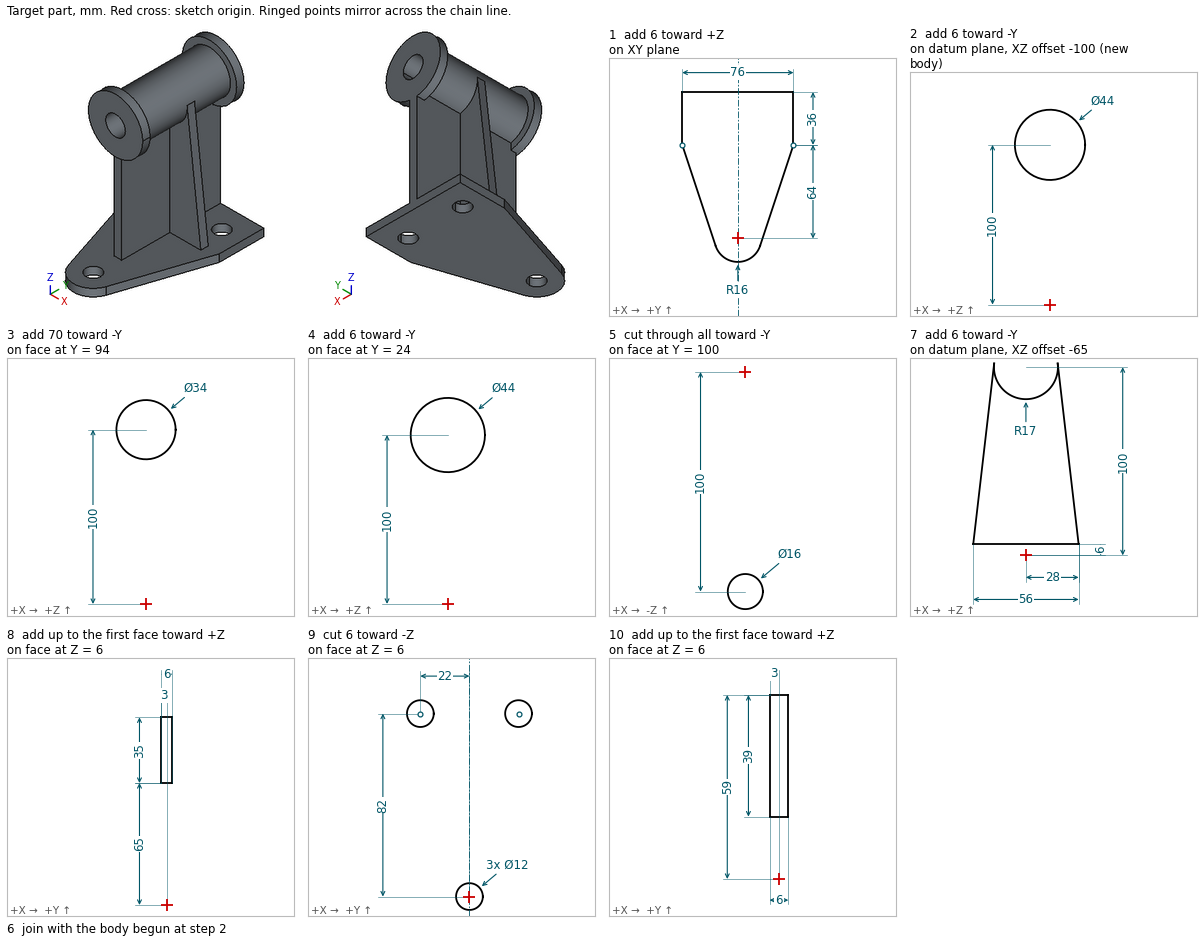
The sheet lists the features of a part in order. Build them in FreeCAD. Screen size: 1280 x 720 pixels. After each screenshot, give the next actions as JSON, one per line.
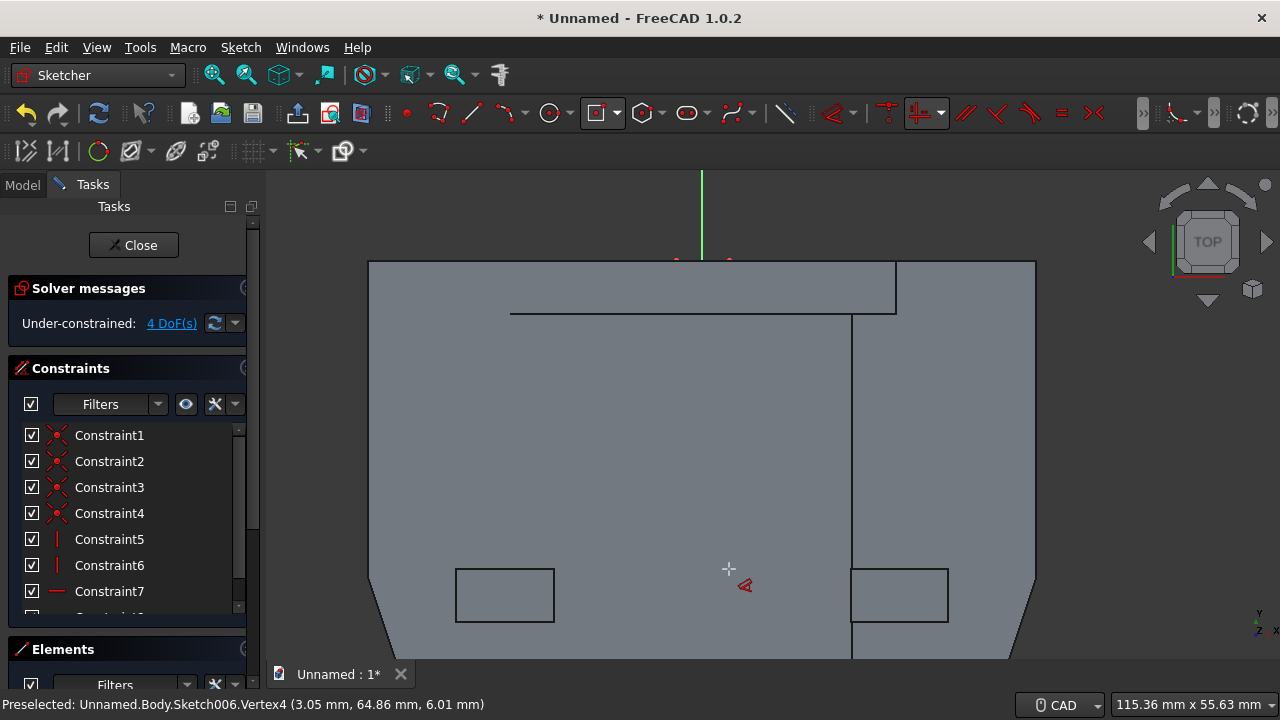
{"action": "scroll", "coordinate": [692, 570], "scroll_direction": "up", "scroll_amount": 2}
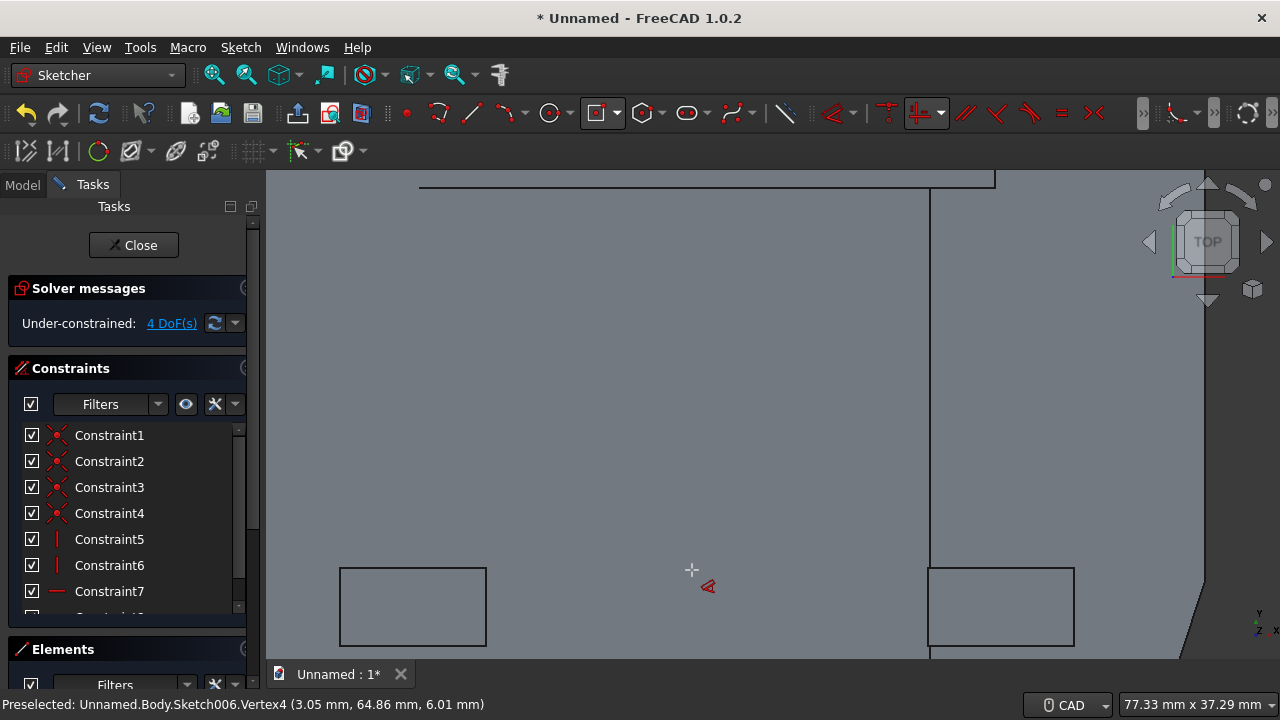
{"action": "left_click", "coordinate": [692, 570]}
{"action": "left_click", "coordinate": [689, 604]}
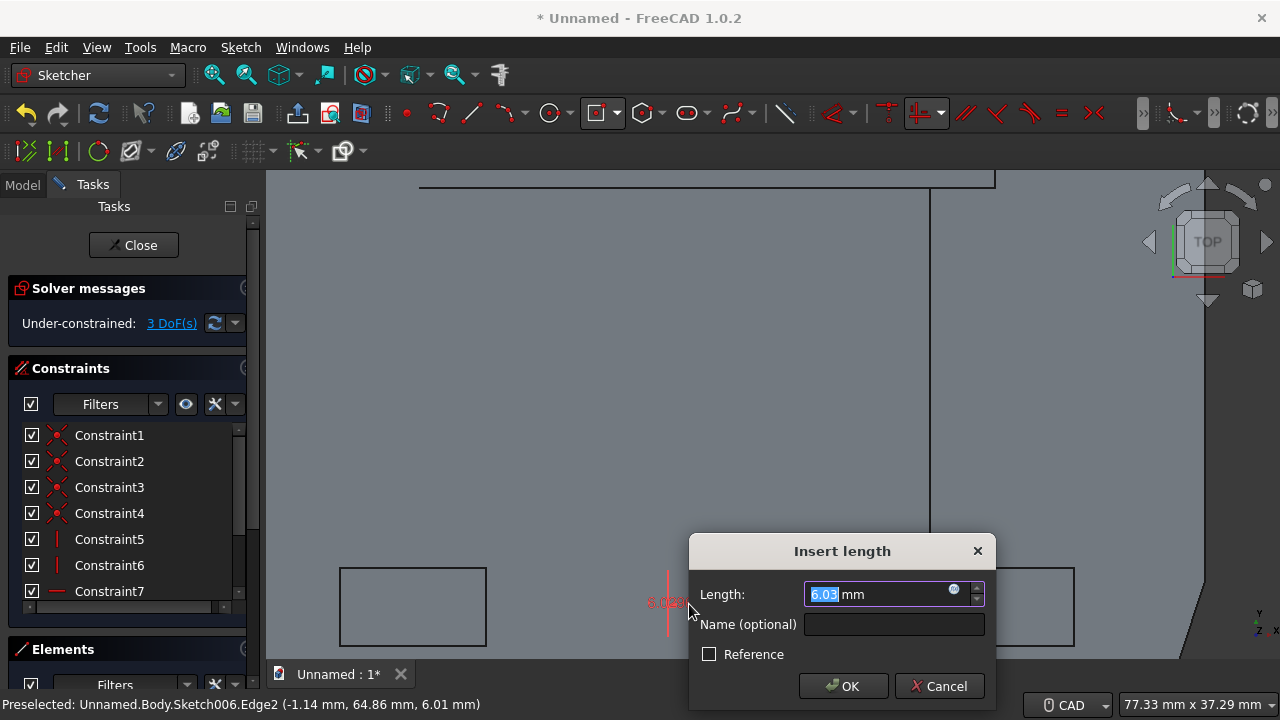
{"action": "type", "text": "6"}
{"action": "key", "text": "Return"}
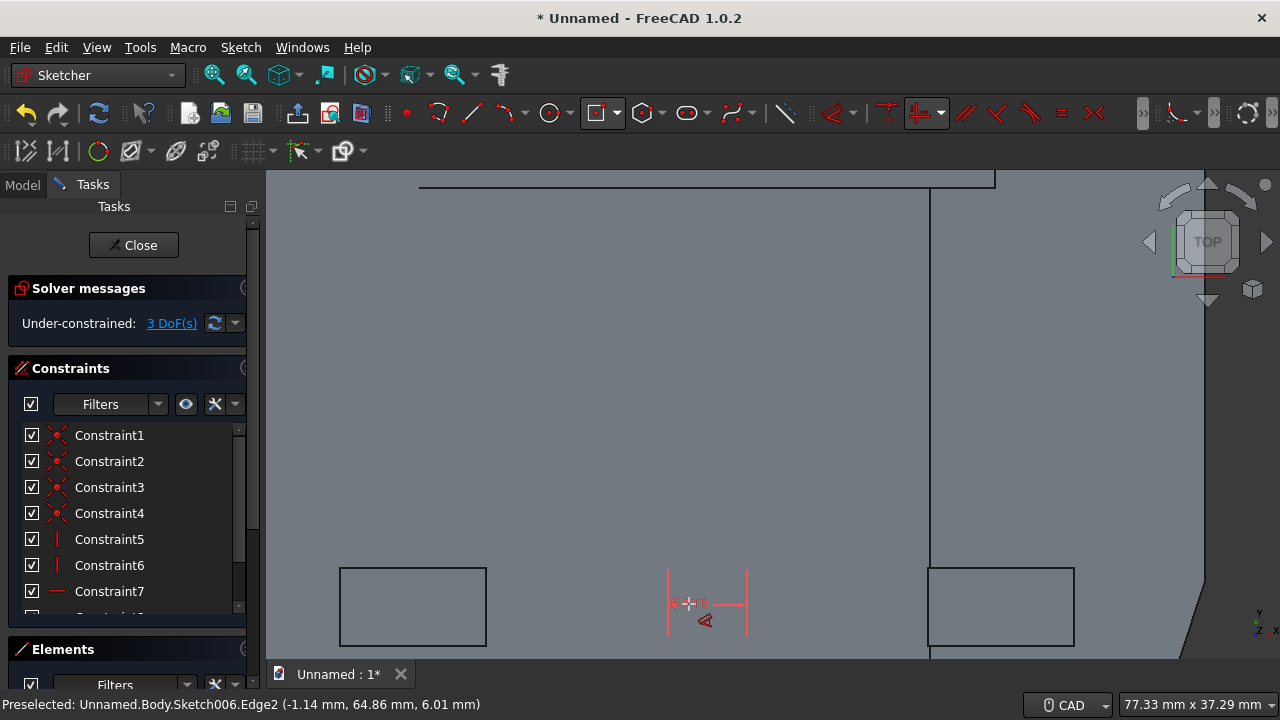
{"action": "left_click", "coordinate": [668, 248]}
{"action": "left_click", "coordinate": [634, 384]}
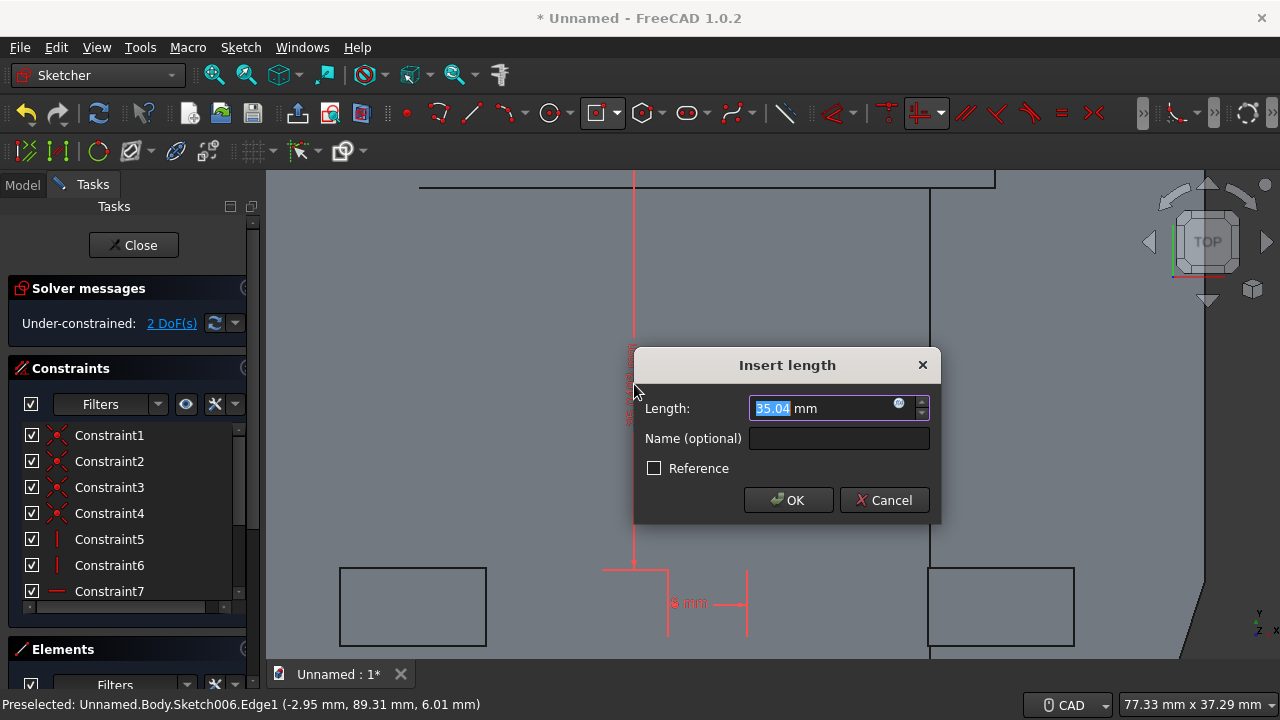
{"action": "type", "text": "35"}
{"action": "key", "text": "Return"}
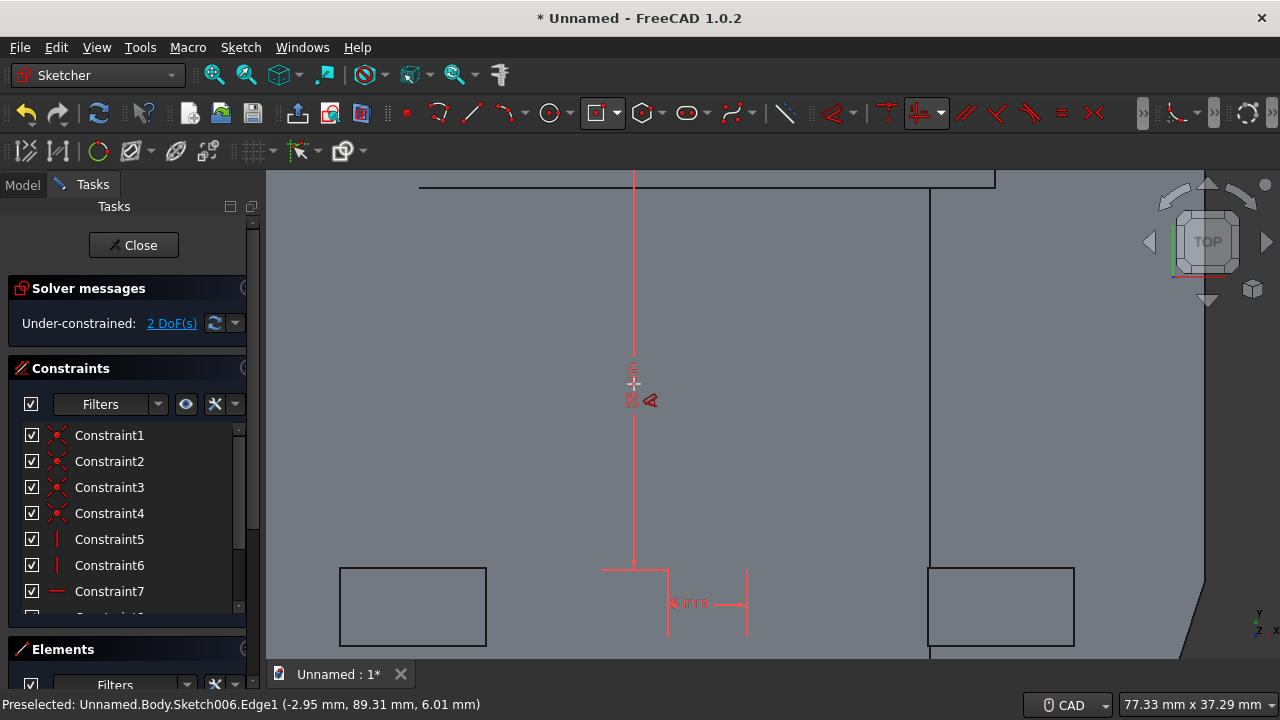
{"action": "scroll", "coordinate": [699, 569], "scroll_direction": "down", "scroll_amount": 2}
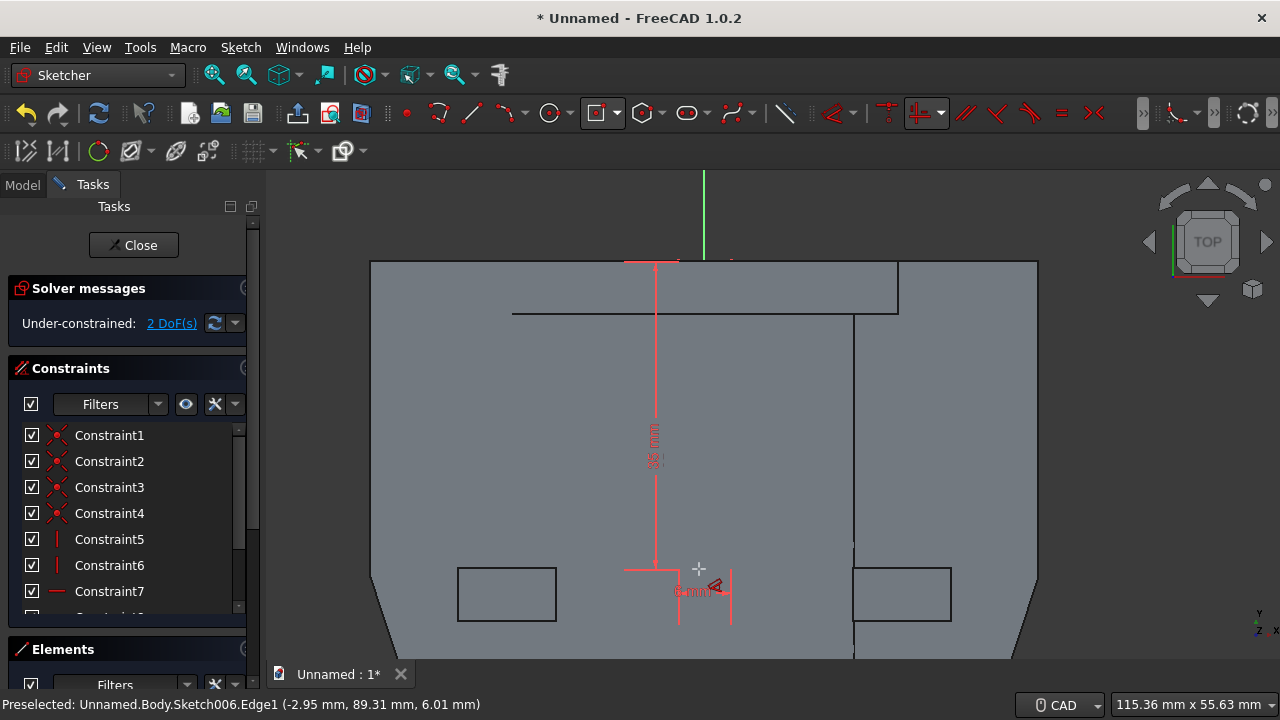
{"action": "scroll", "coordinate": [679, 262], "scroll_direction": "up", "scroll_amount": 3}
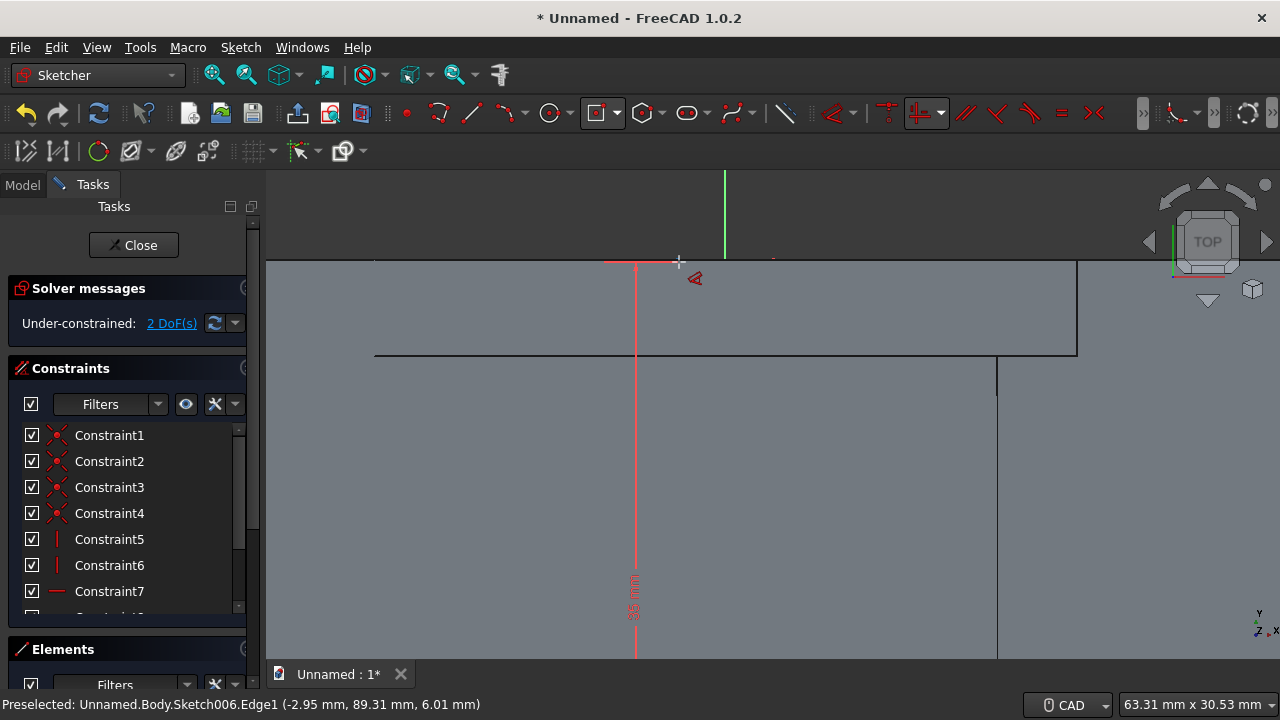
{"action": "left_click", "coordinate": [678, 262]}
{"action": "left_click", "coordinate": [701, 228]}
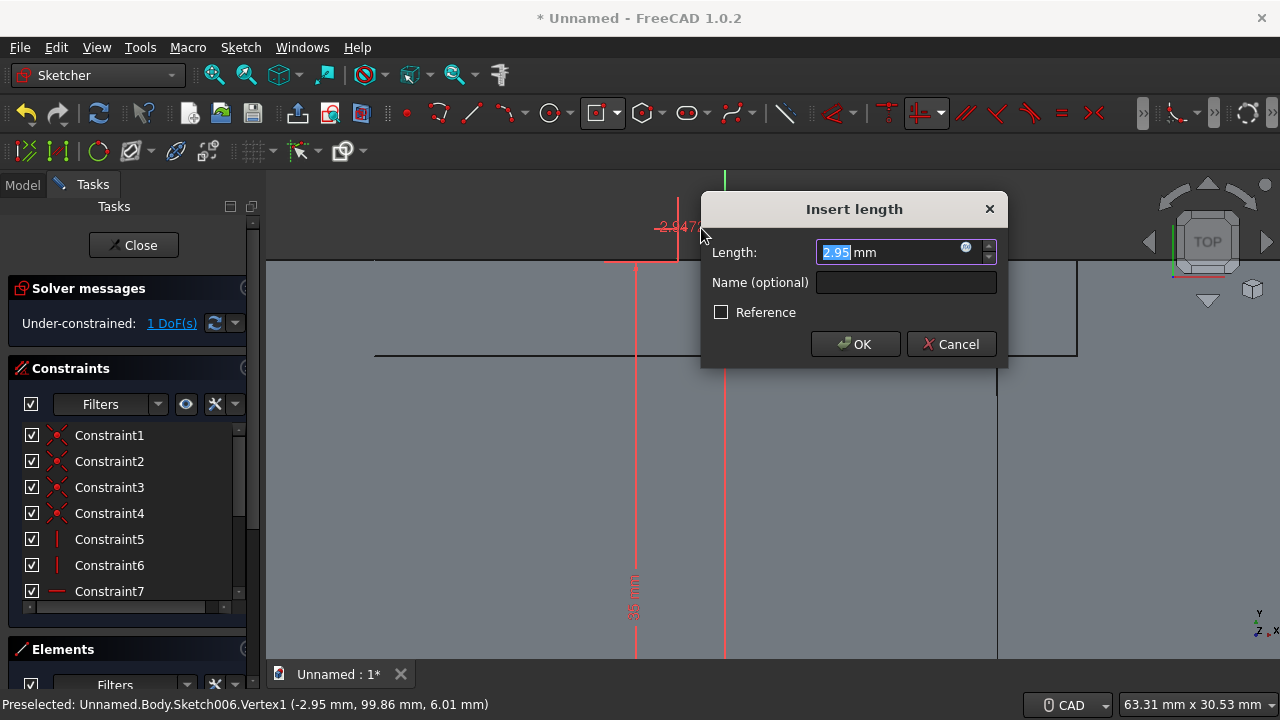
{"action": "type", "text": "3"}
{"action": "key", "text": "Return"}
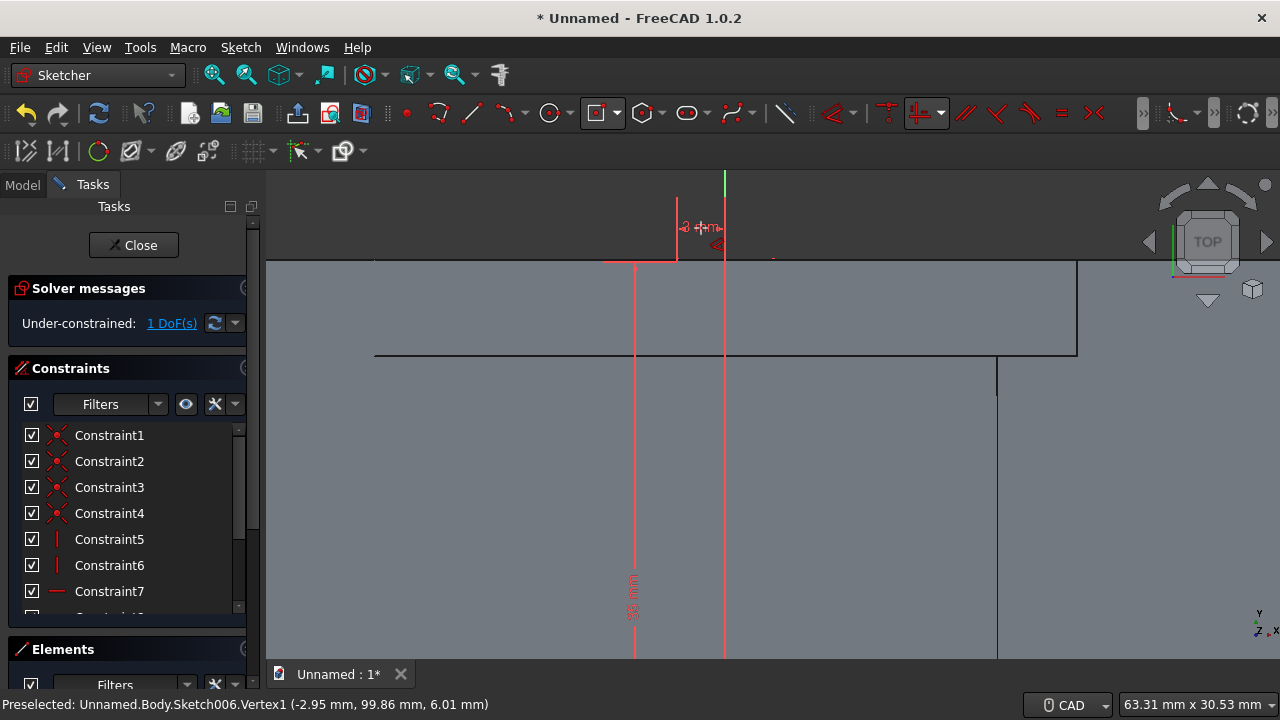
{"action": "scroll", "coordinate": [679, 262], "scroll_direction": "down", "scroll_amount": 3}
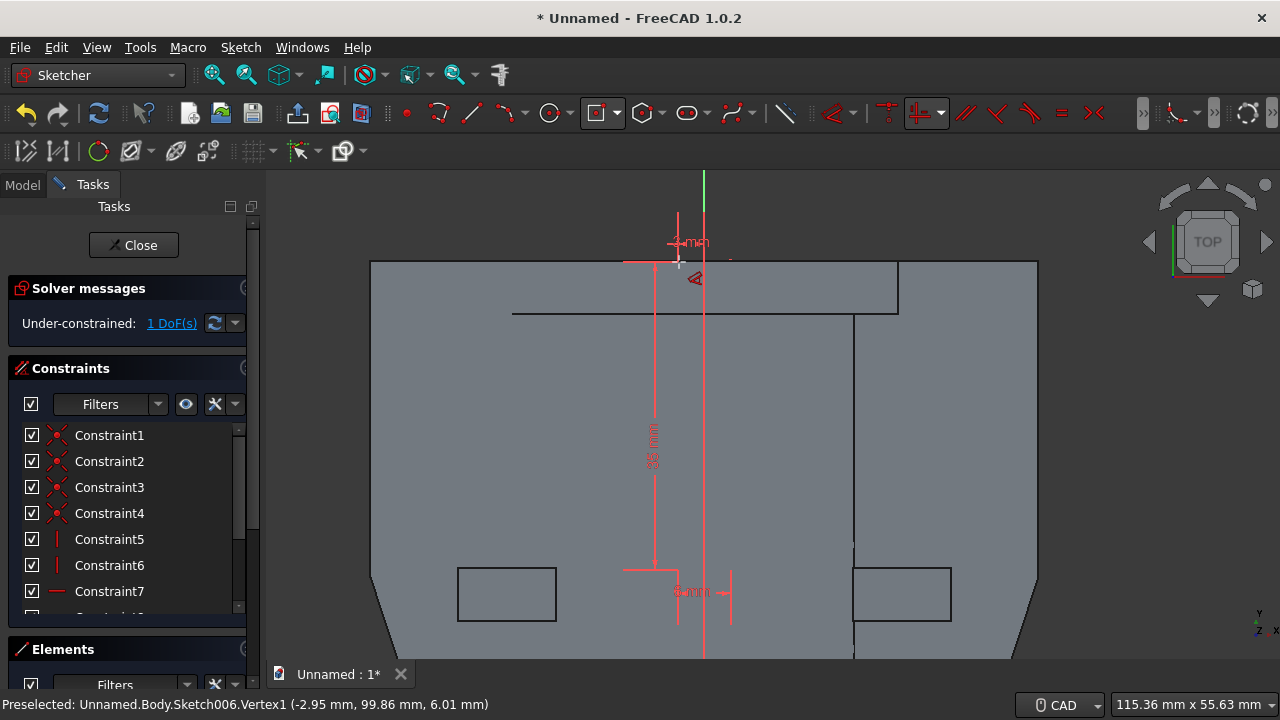
{"action": "left_click", "coordinate": [678, 570]}
{"action": "left_click", "coordinate": [644, 614]}